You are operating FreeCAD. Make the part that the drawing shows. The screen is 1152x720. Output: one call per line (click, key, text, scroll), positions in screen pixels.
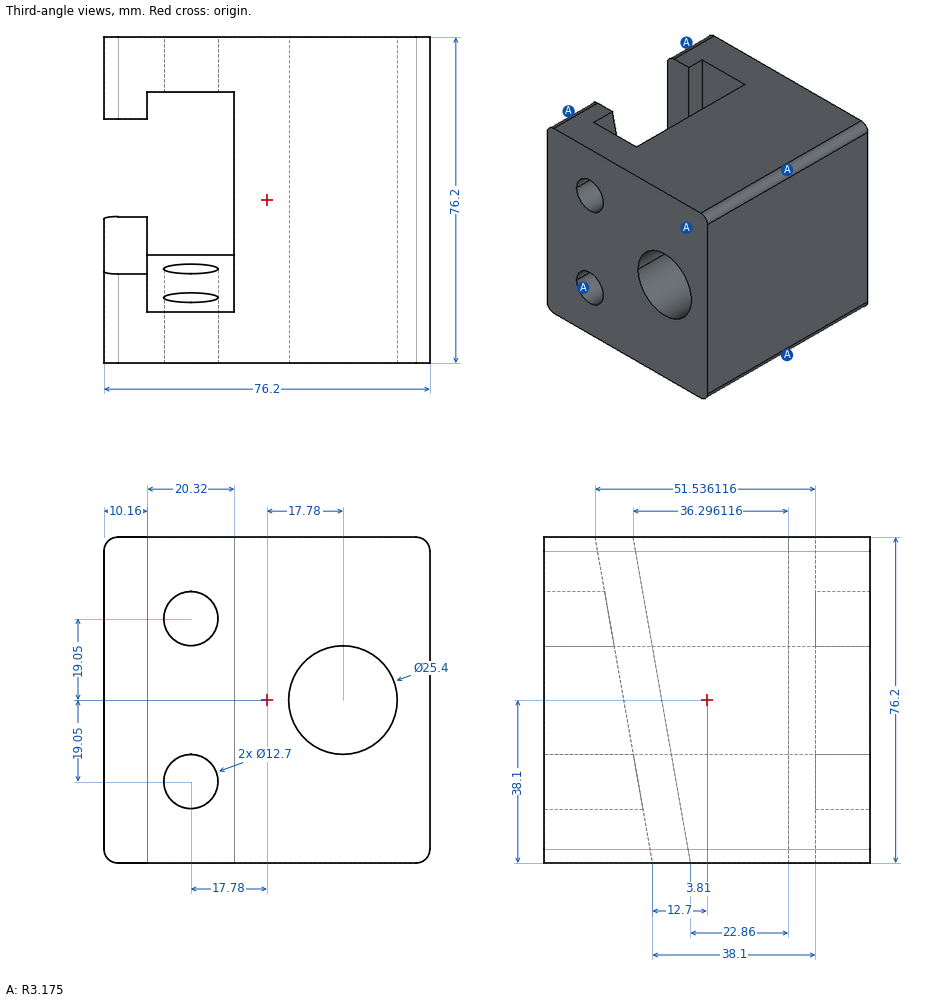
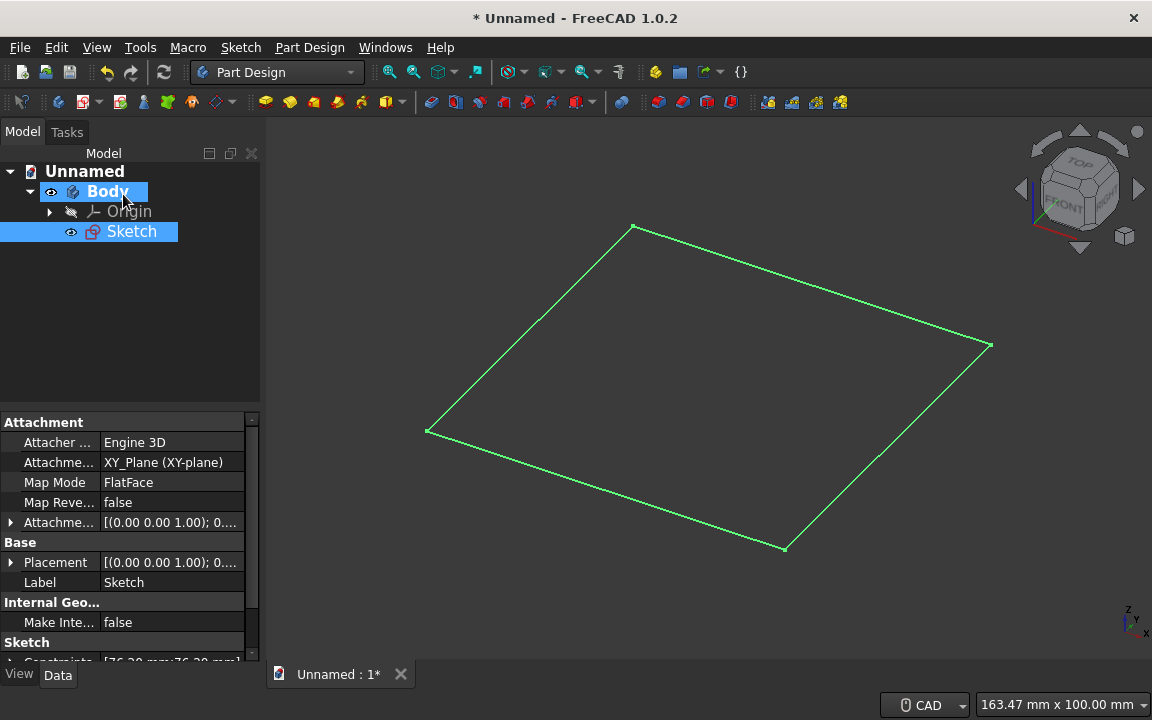
click(266, 102)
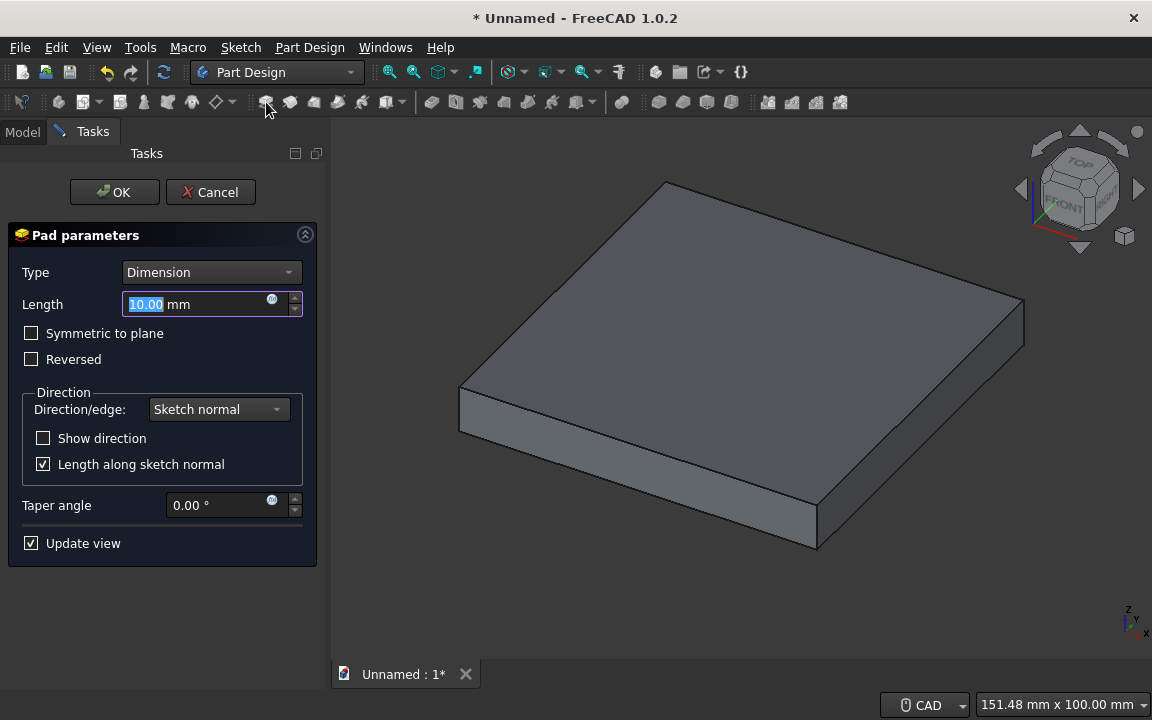
text(76.2)
key(Tab)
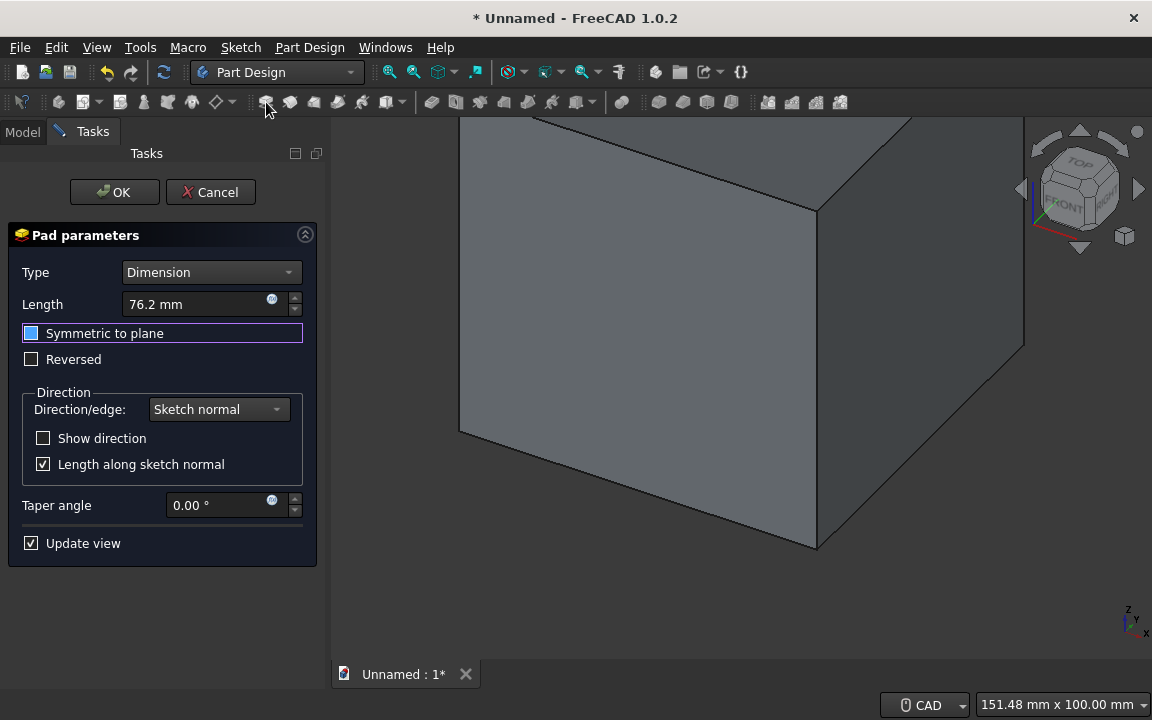
click(30, 333)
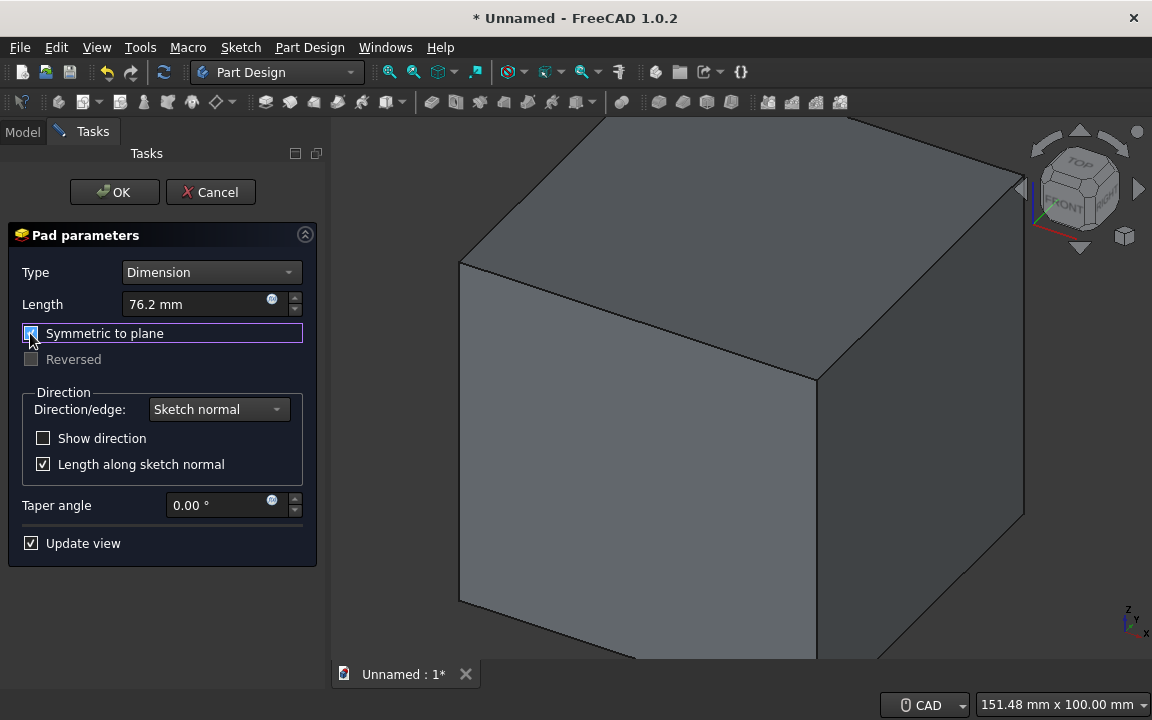
click(115, 192)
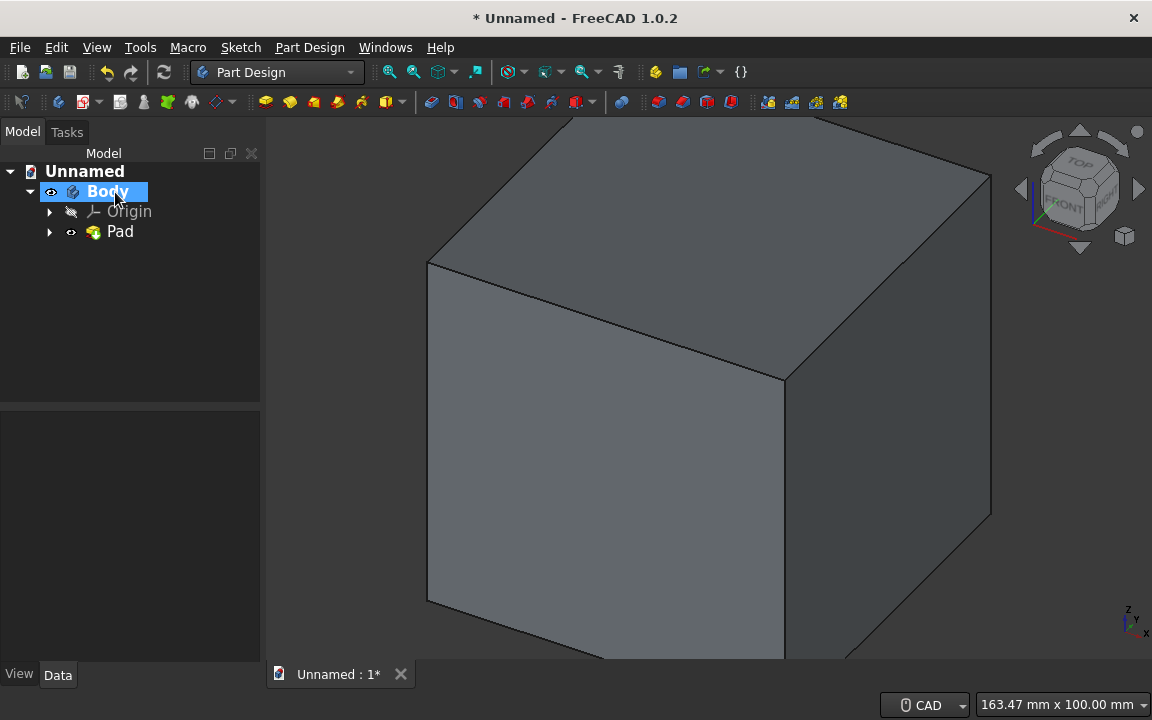
key(v)
key(f)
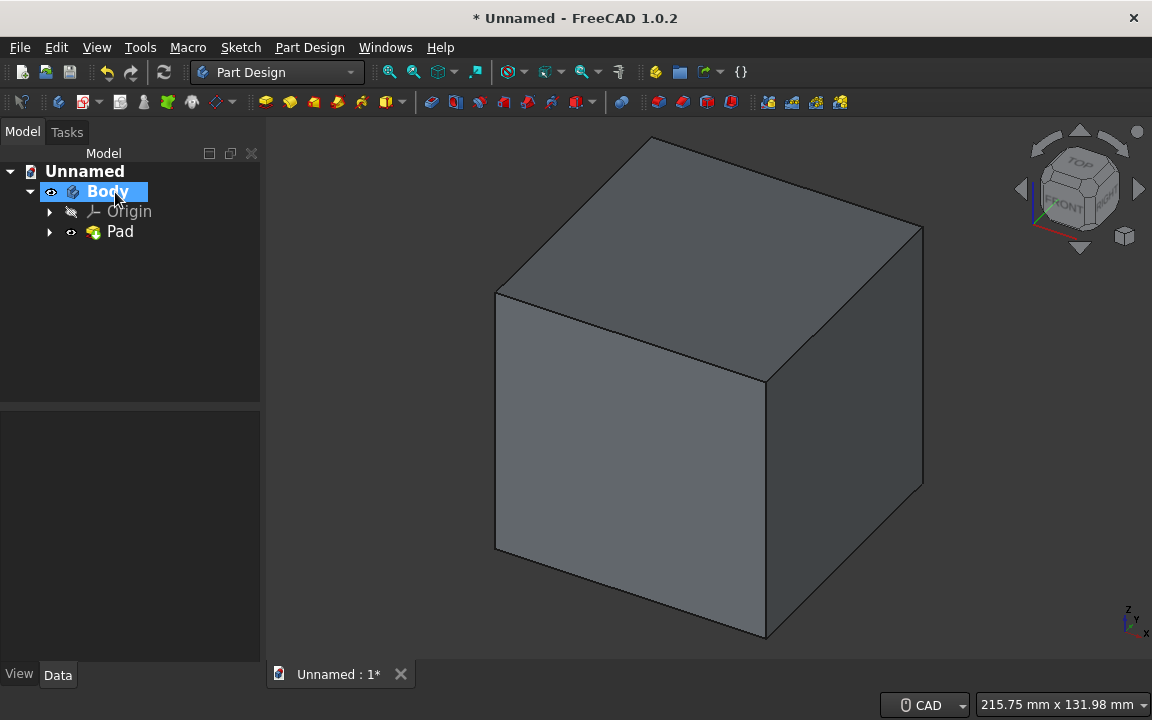
key(6)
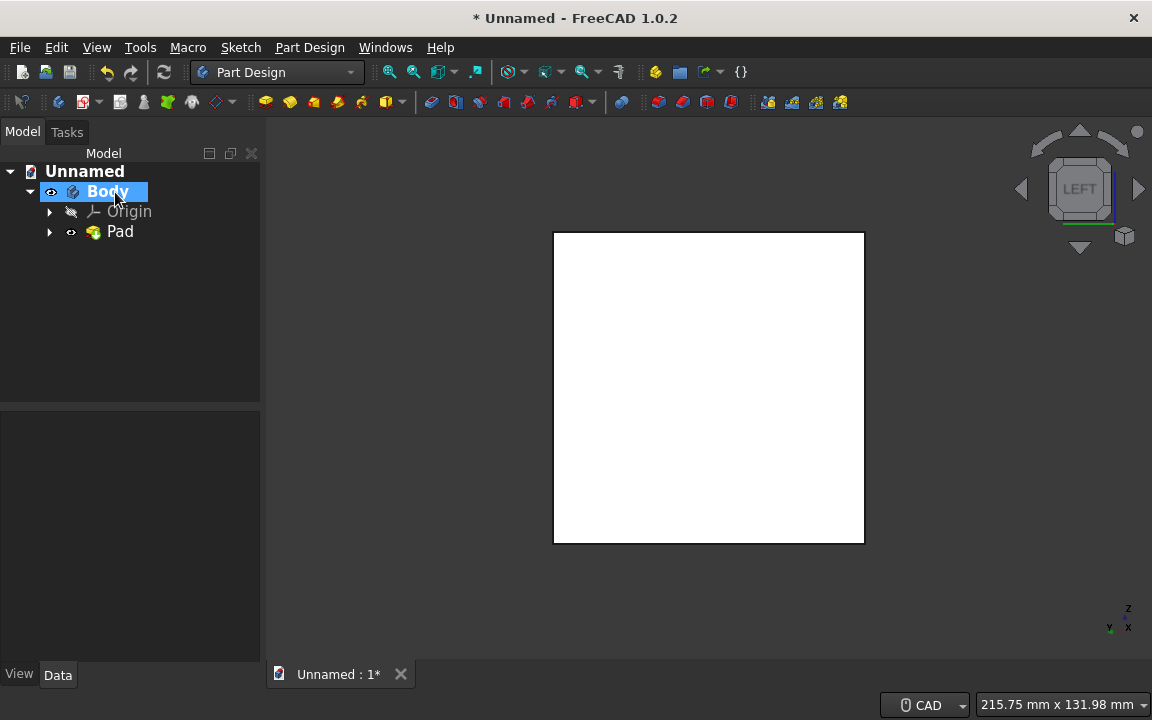
click(709, 387)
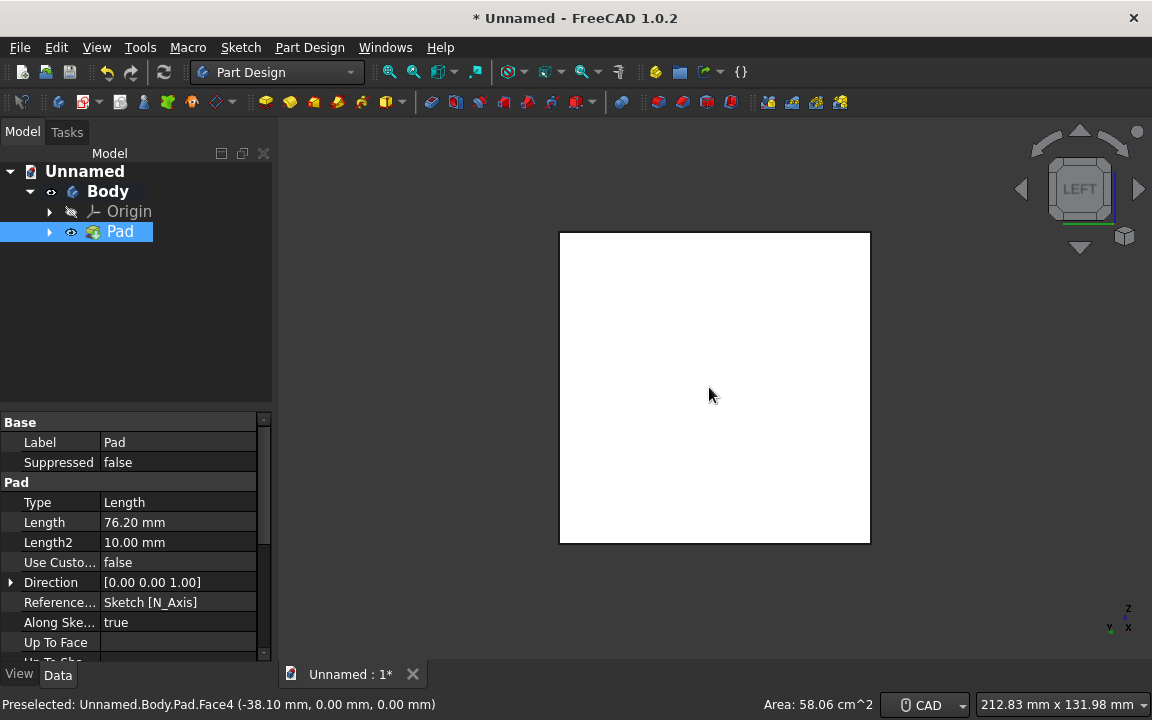
click(84, 102)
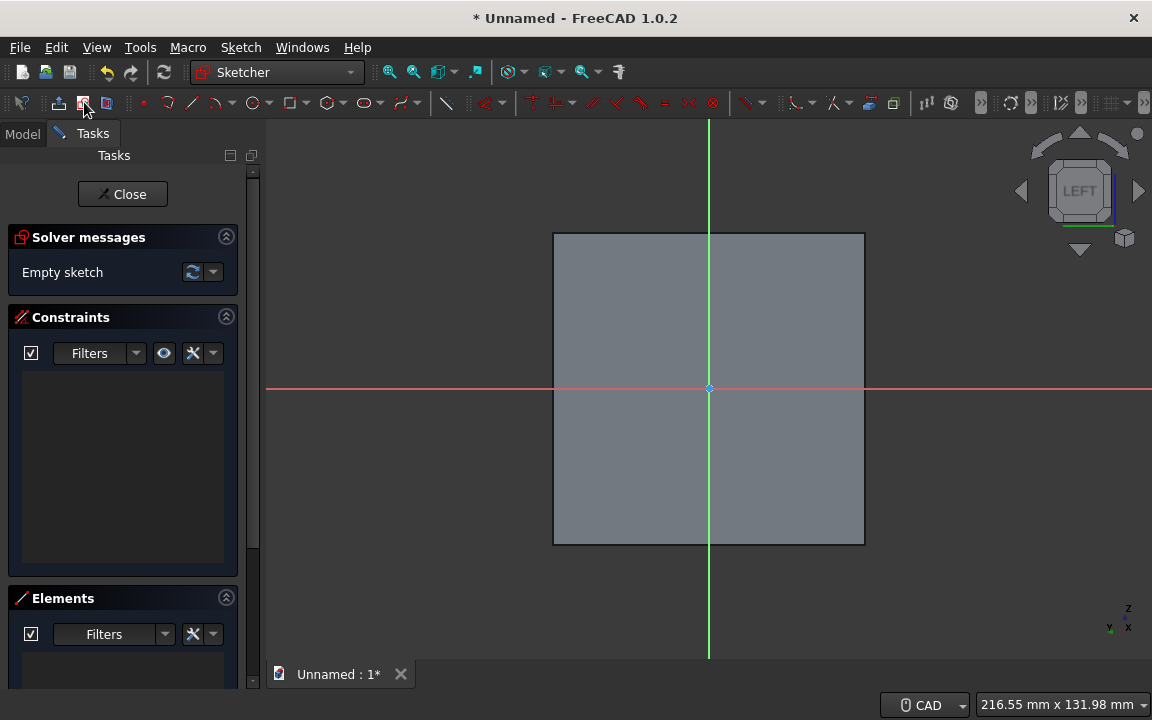
key(g)
key(m)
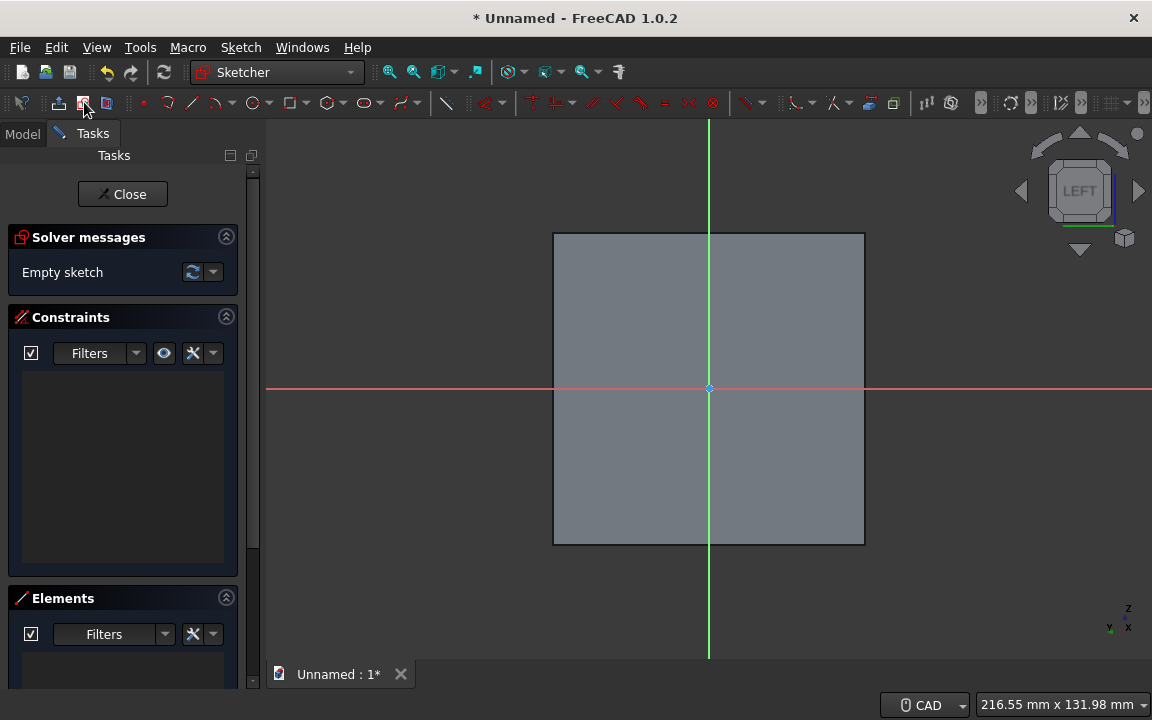
click(725, 545)
click(780, 233)
click(631, 233)
click(631, 545)
click(725, 546)
key(Escape)
key(Escape)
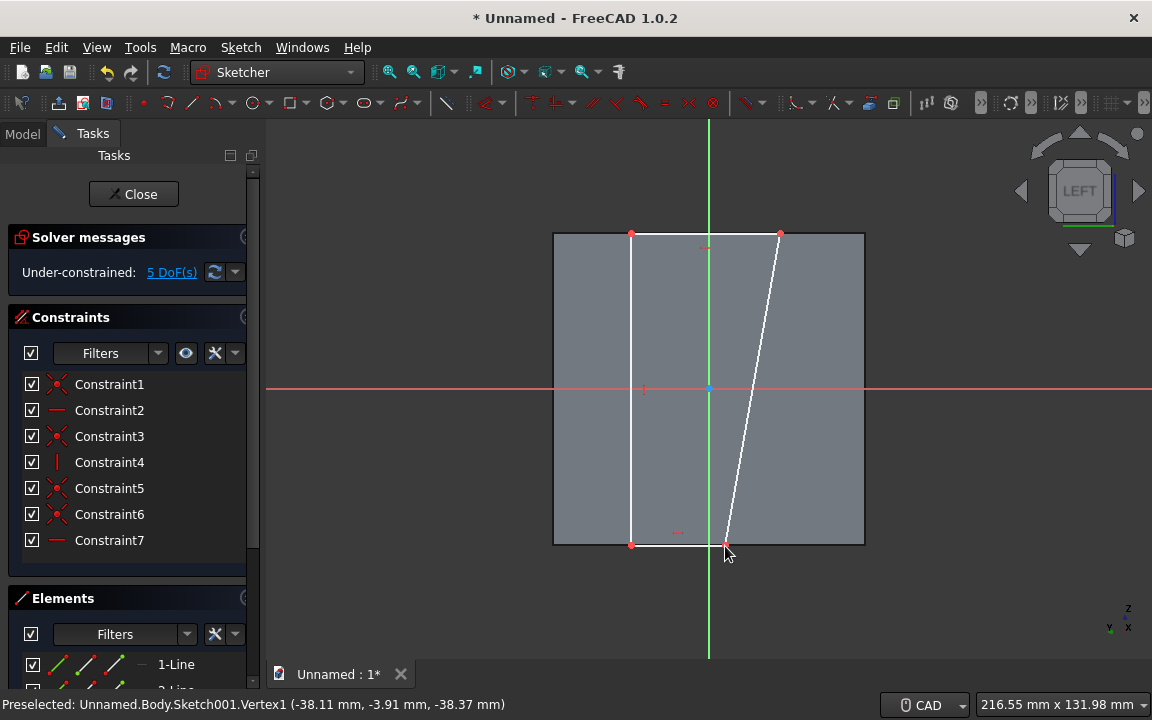
key(d)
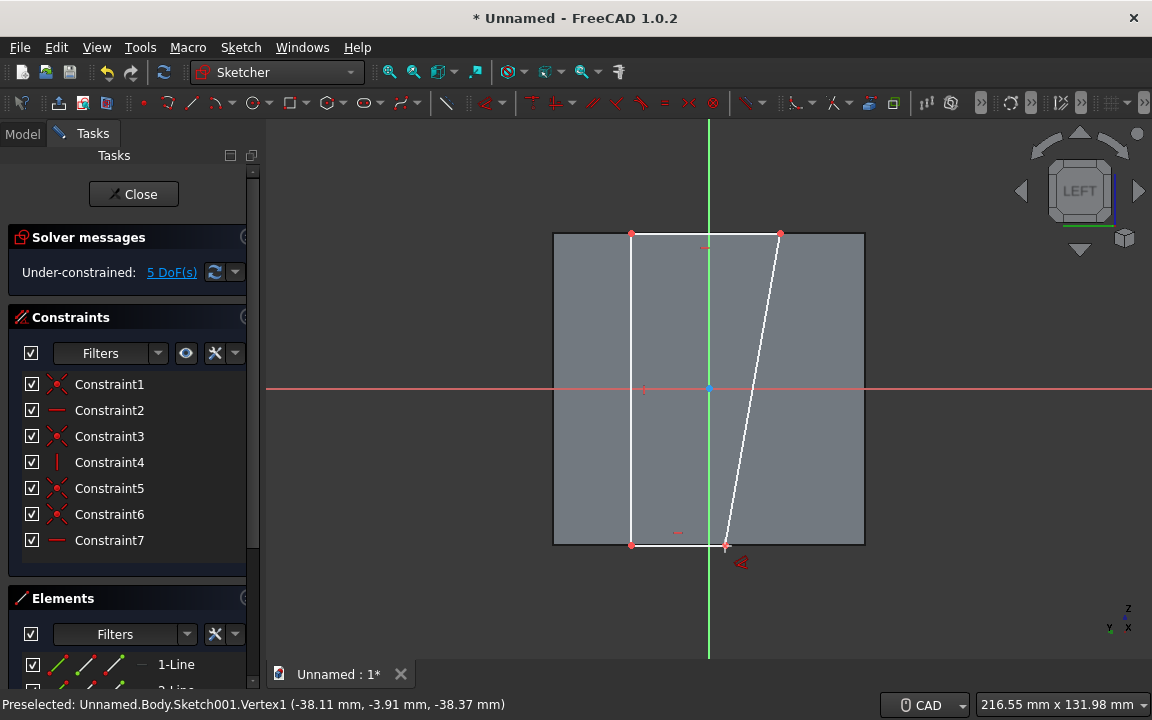
click(631, 328)
click(597, 318)